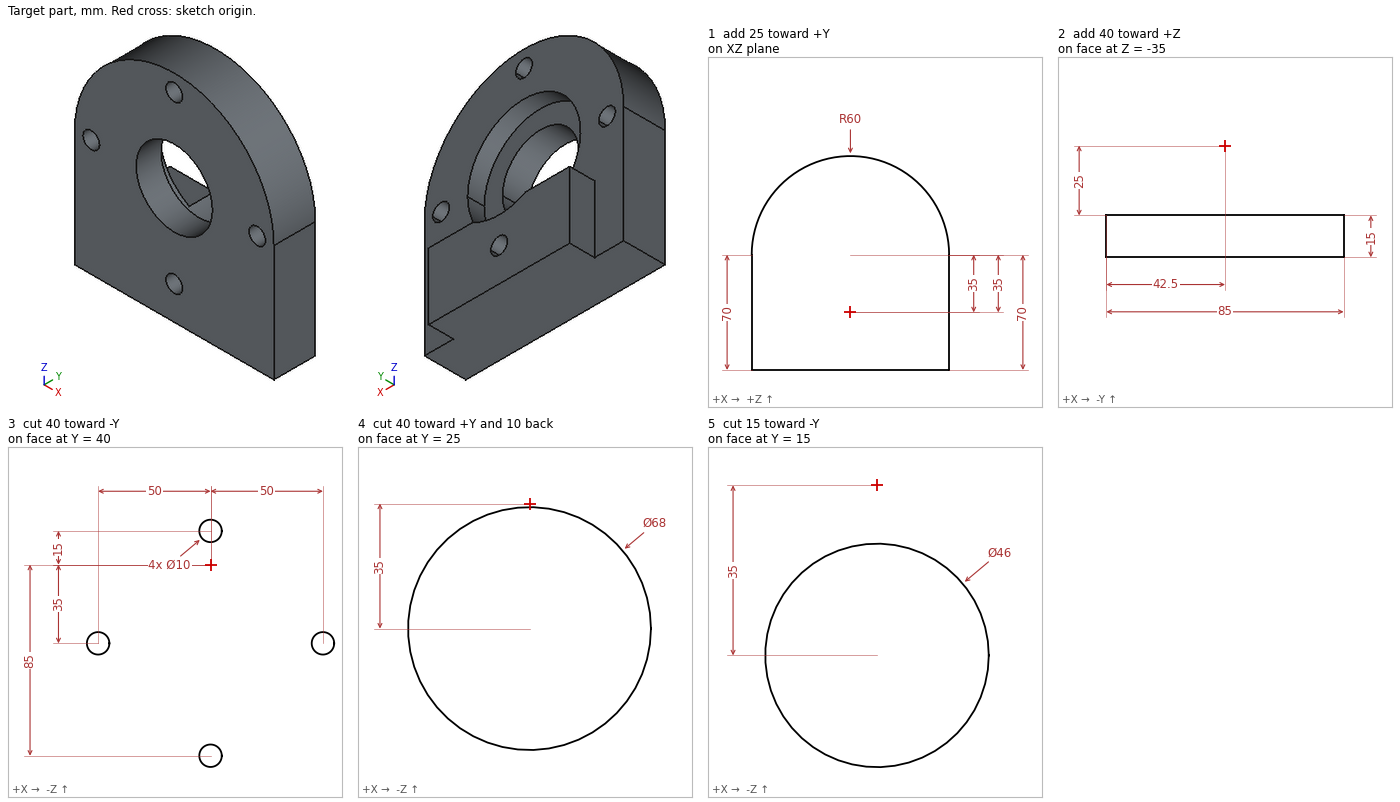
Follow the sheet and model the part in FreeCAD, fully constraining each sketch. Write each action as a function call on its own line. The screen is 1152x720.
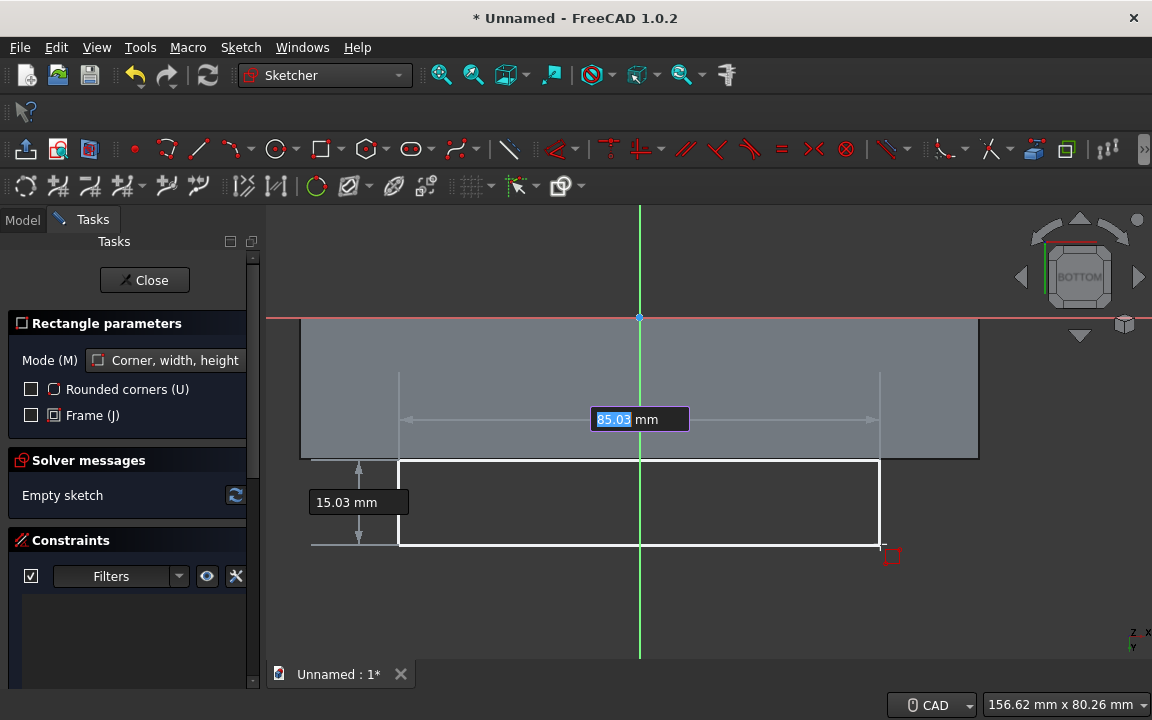
text(85)
key(Tab)
text(15)
key(Return)
key(Escape)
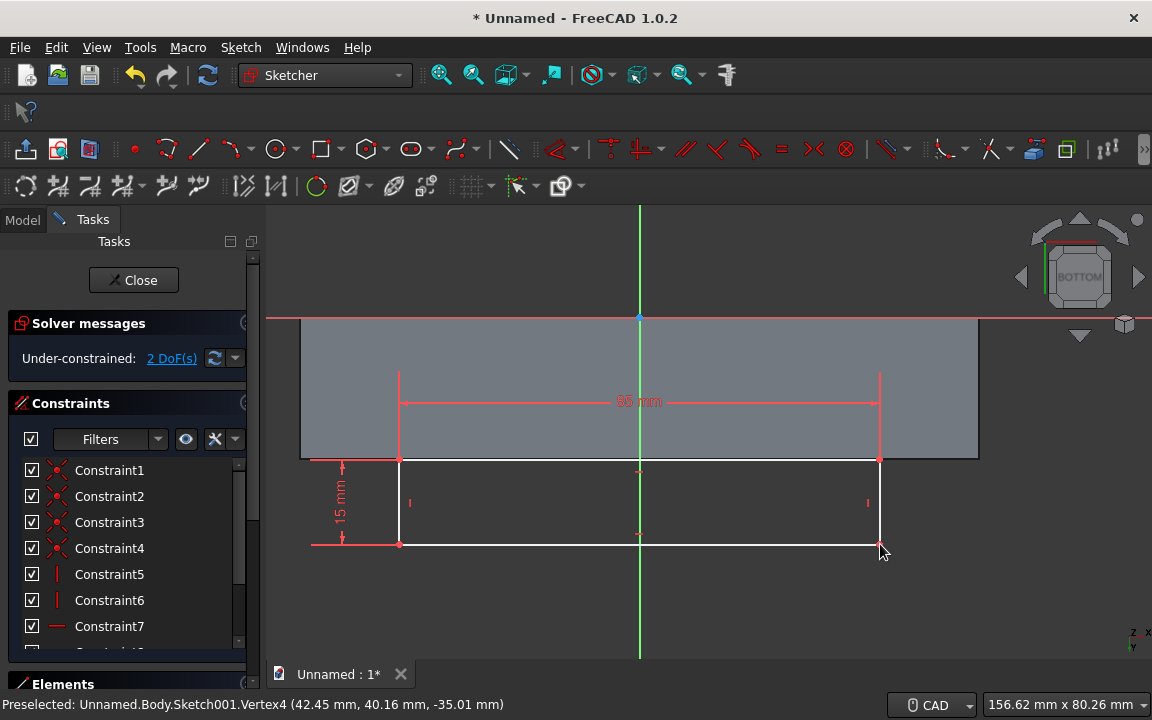
key(d)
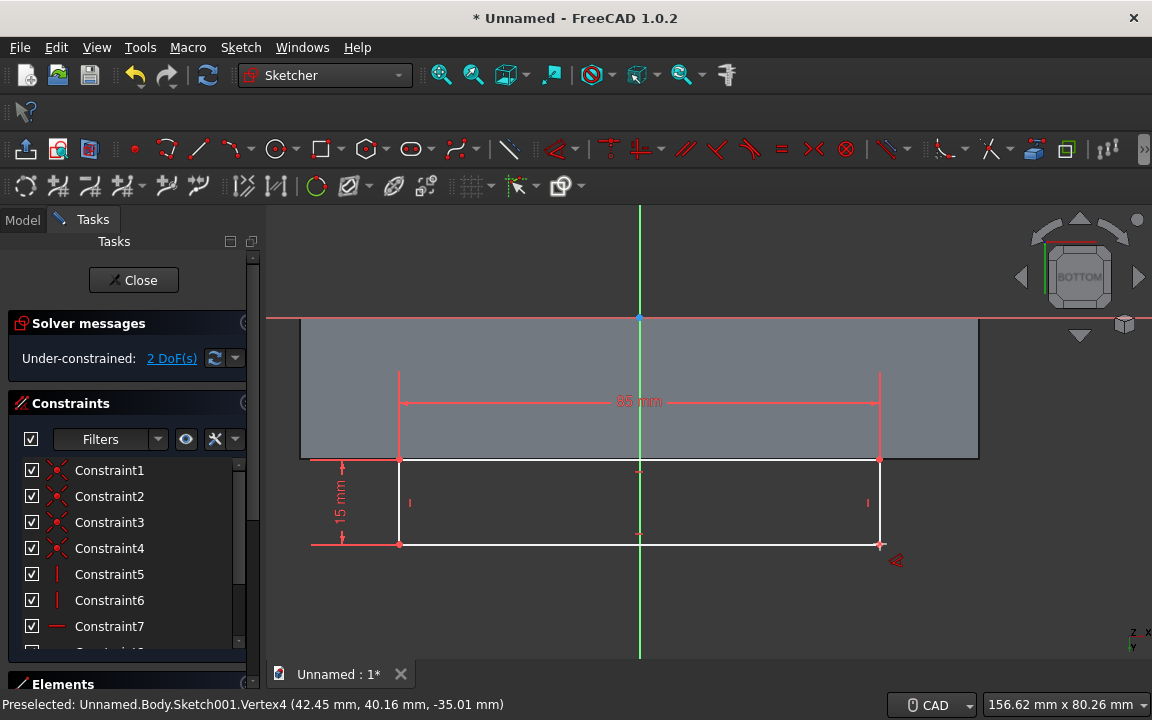
click(399, 460)
click(365, 389)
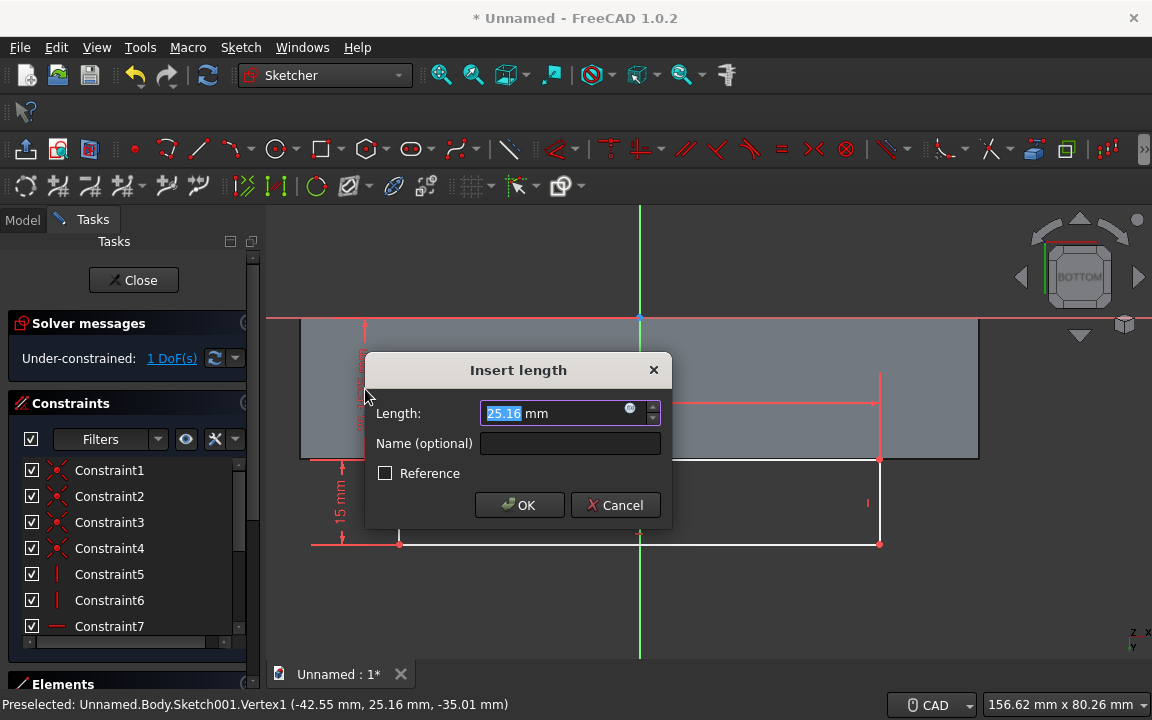
text(25)
key(Return)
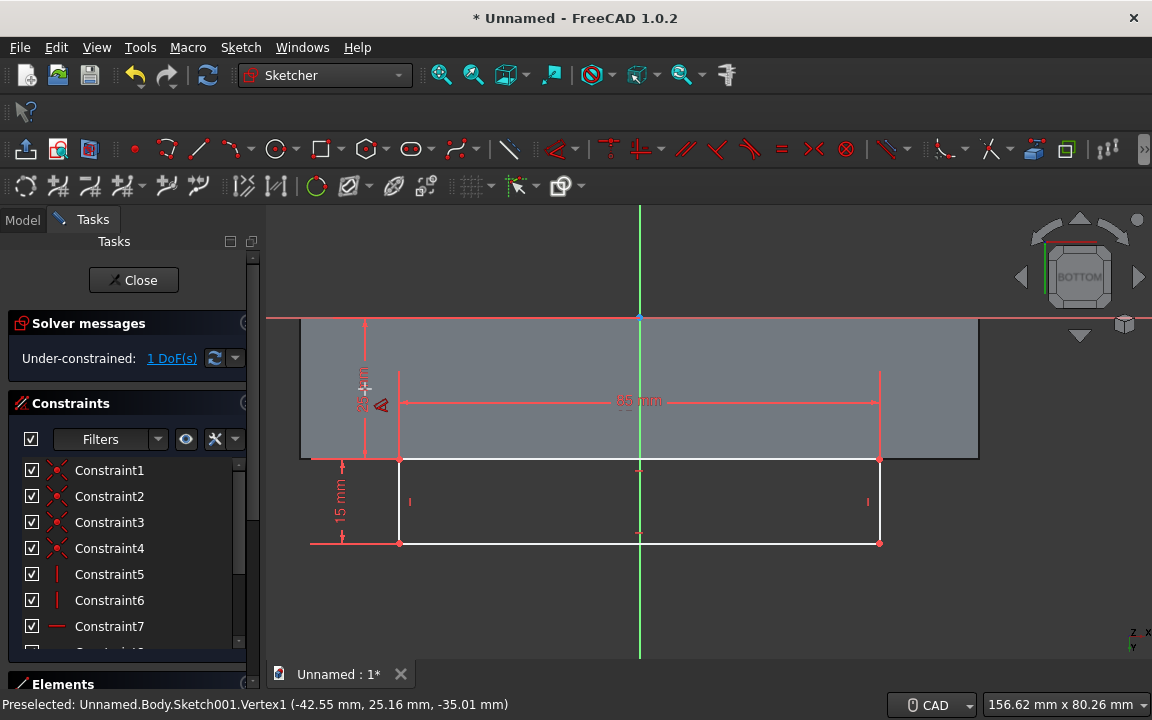
click(399, 459)
click(519, 284)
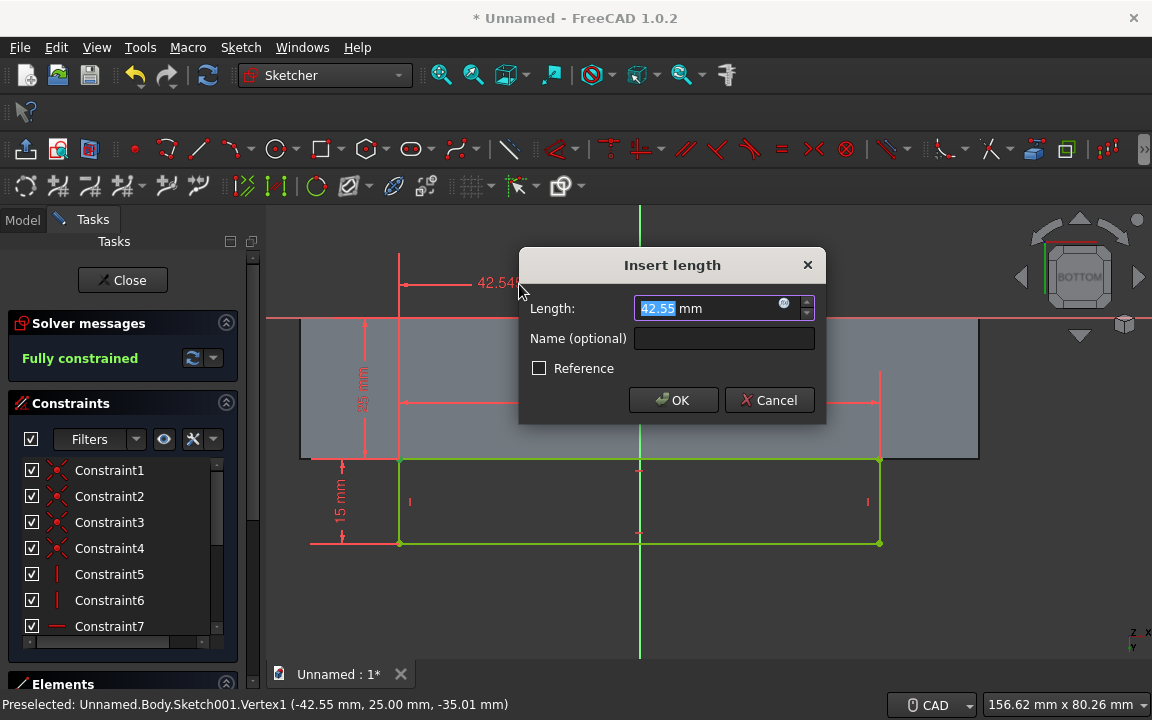
text(42.5)
key(Return)
key(Escape)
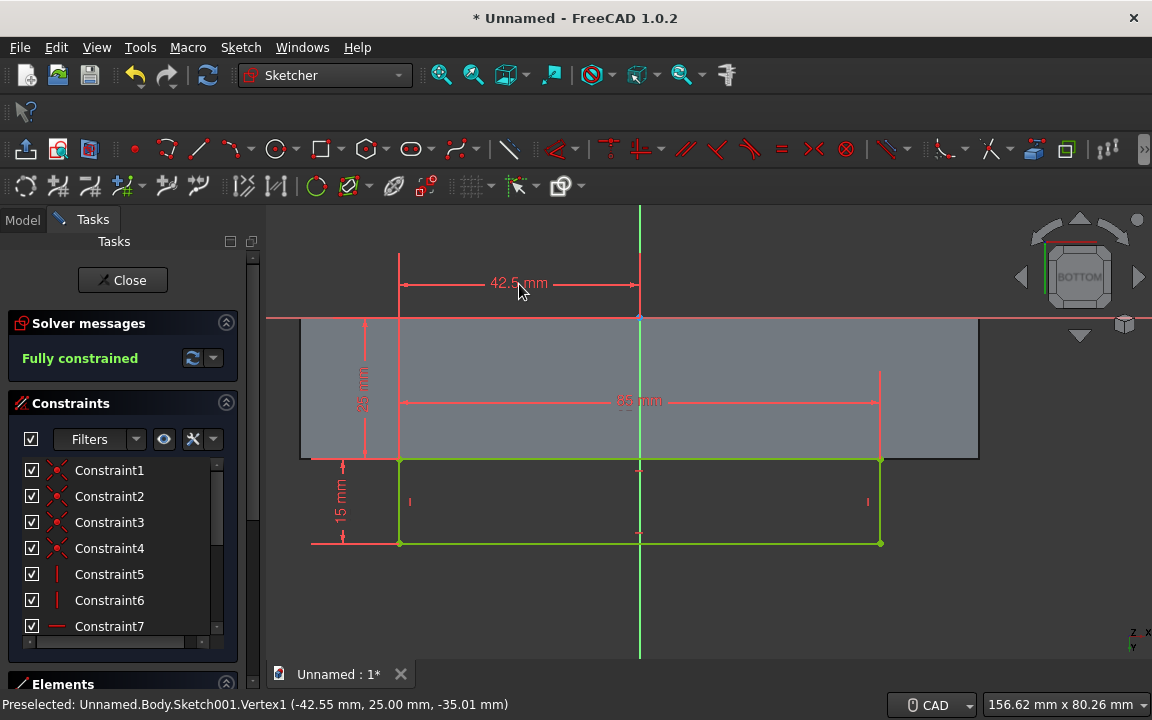
click(123, 280)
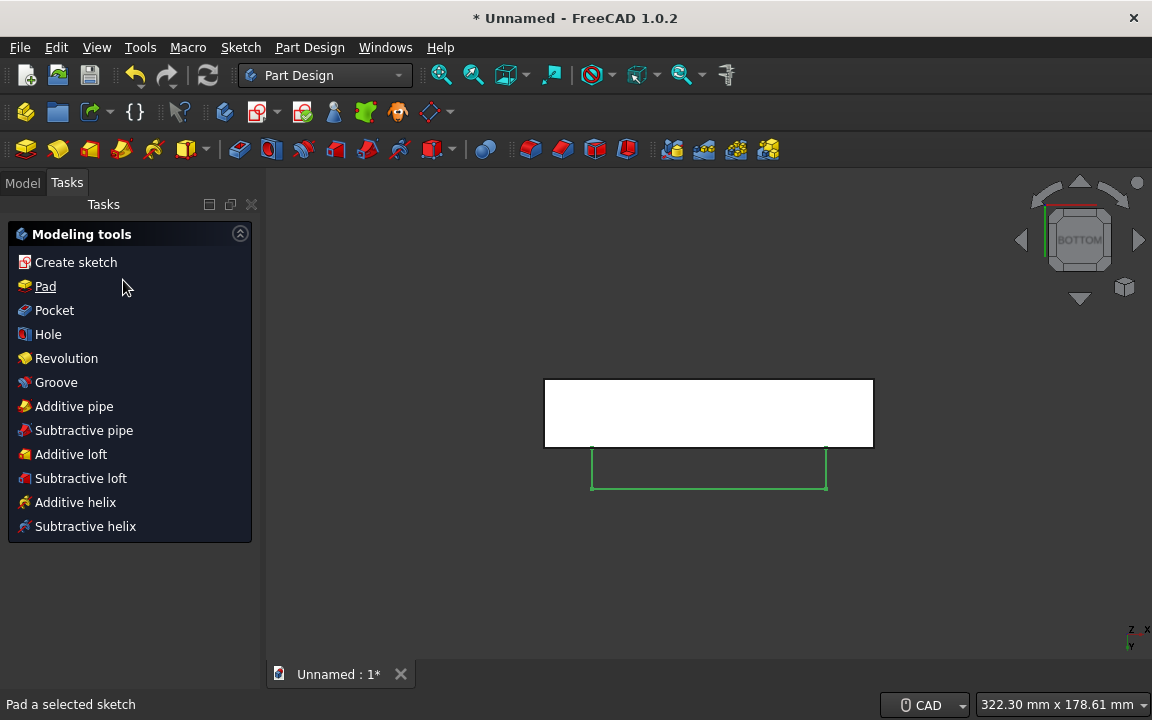
click(26, 150)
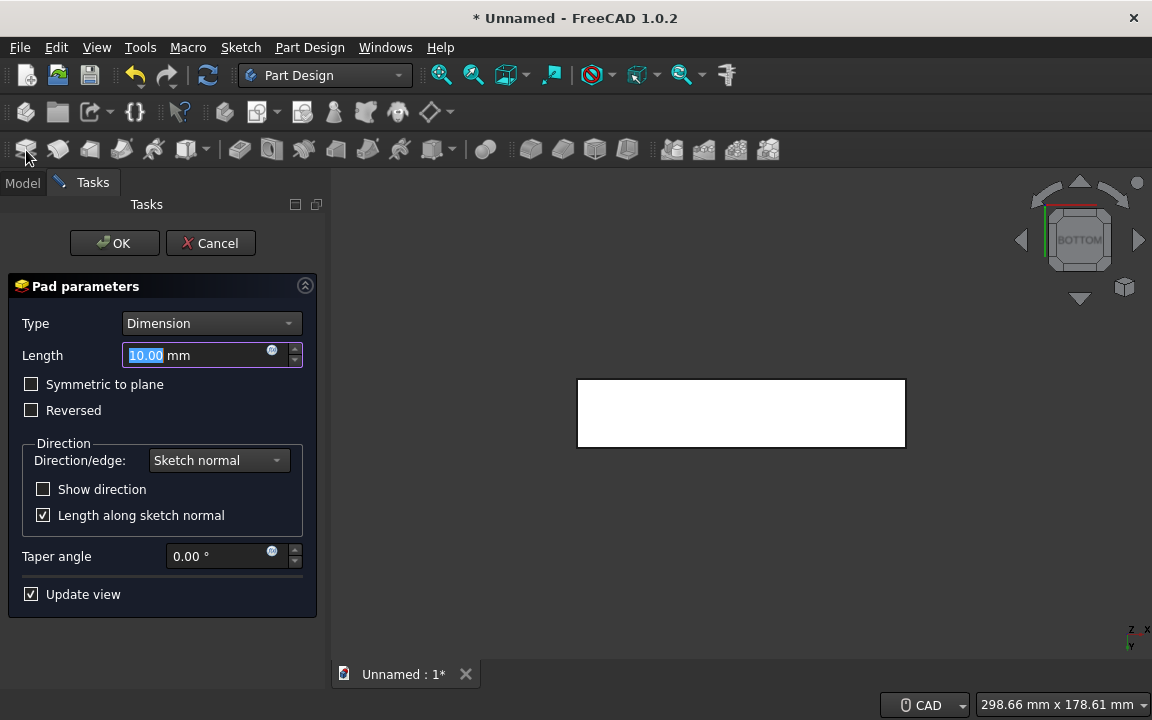
text(40)
key(Tab)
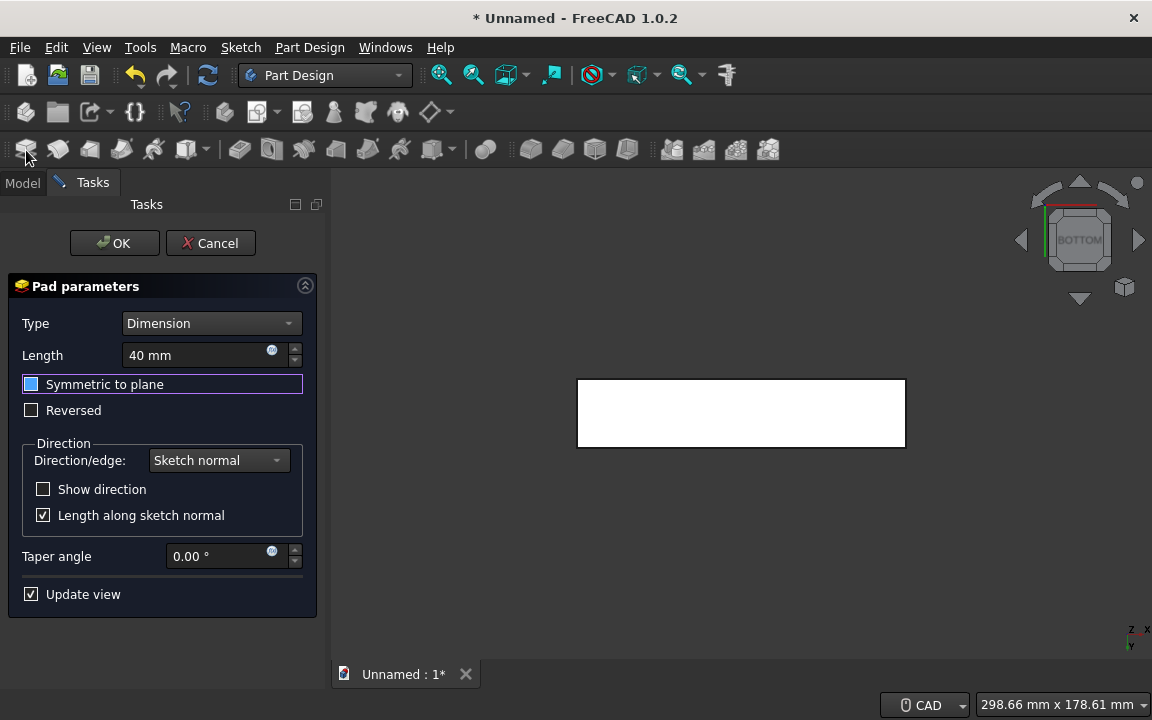
click(30, 410)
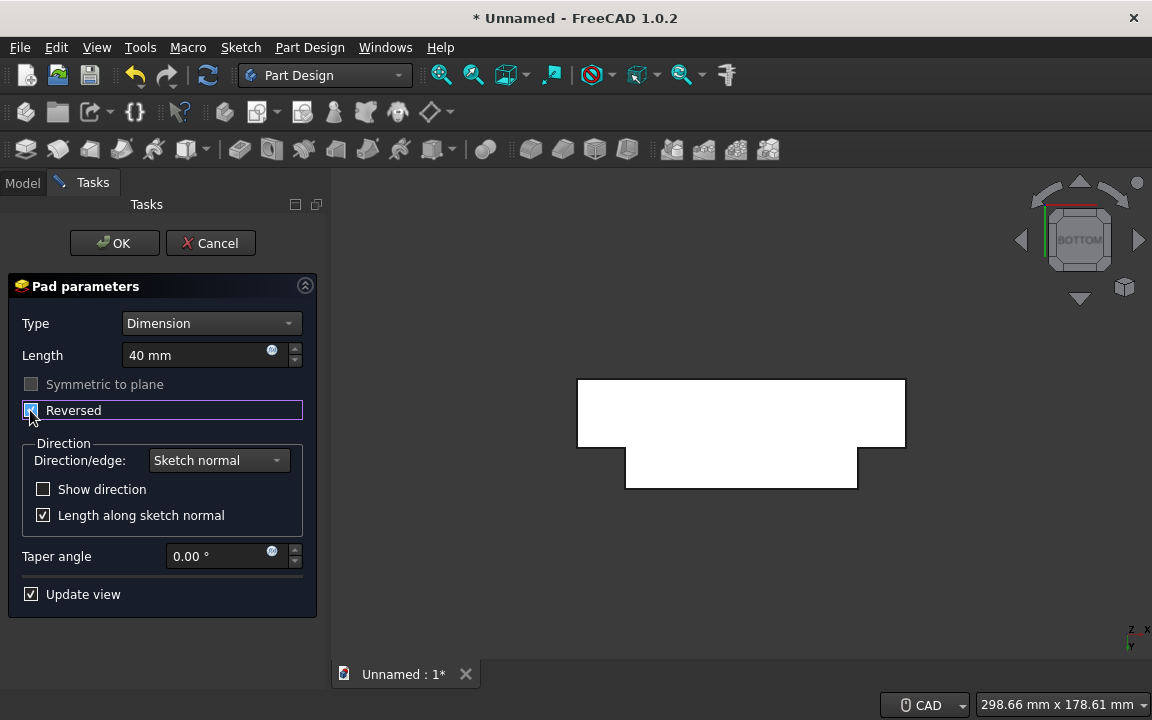
click(115, 243)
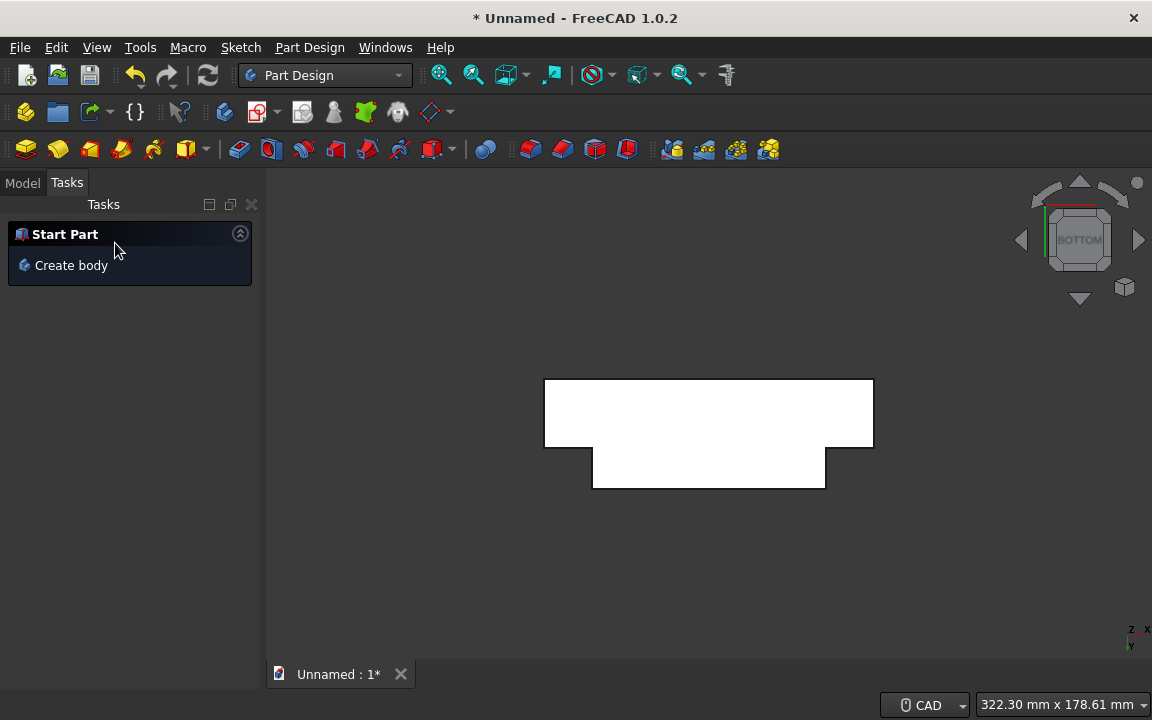
key(v)
key(f)